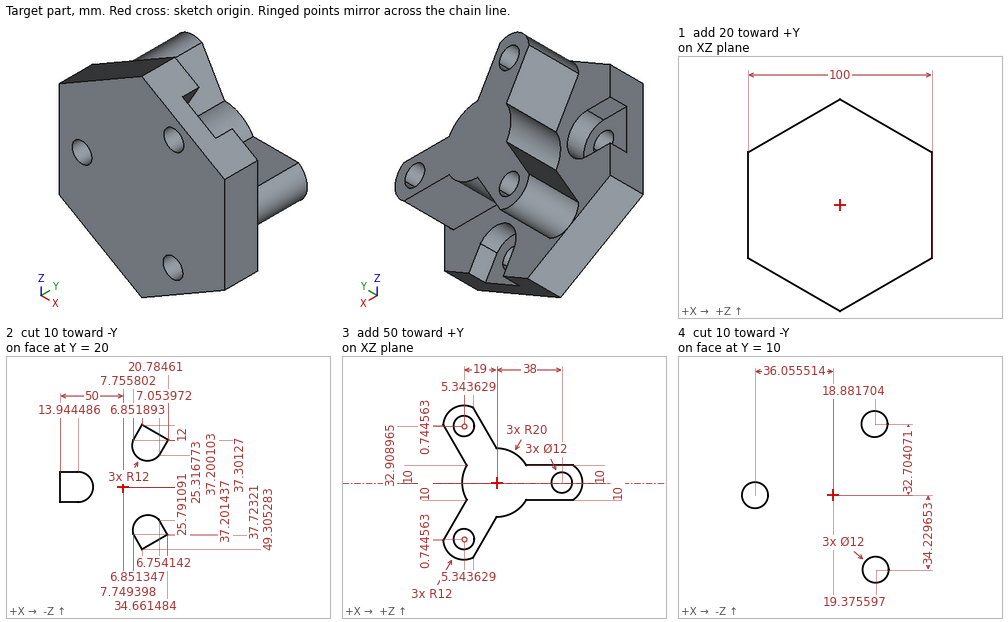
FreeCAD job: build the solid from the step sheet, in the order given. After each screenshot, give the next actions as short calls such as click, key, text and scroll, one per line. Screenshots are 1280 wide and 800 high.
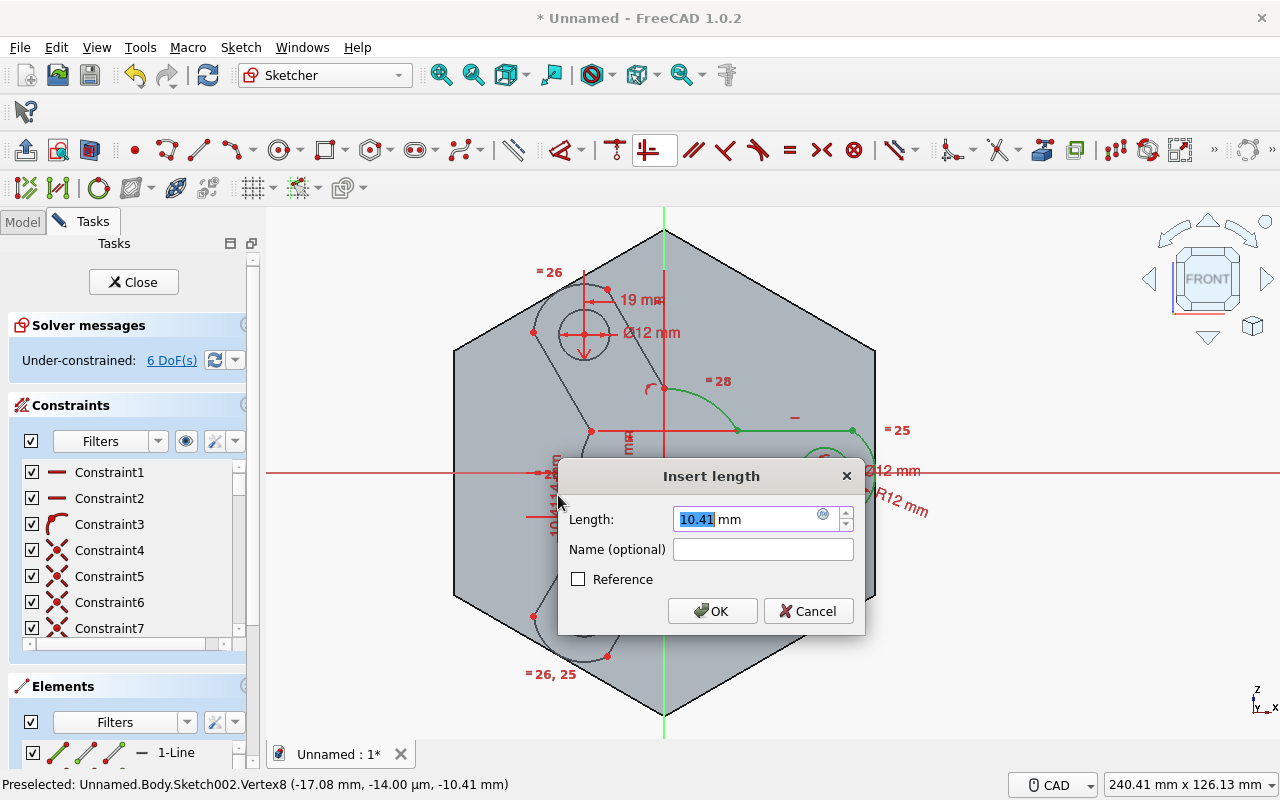
text(10)
key(Return)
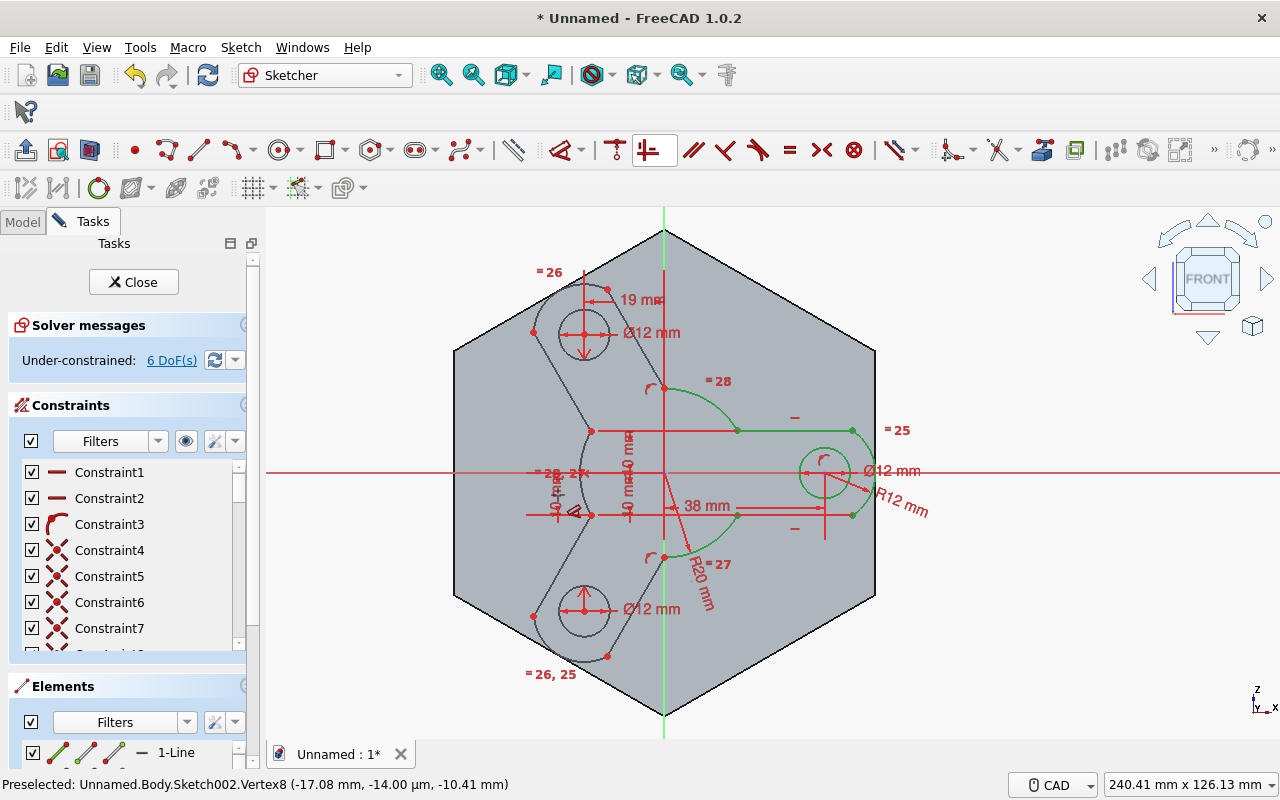
click(591, 432)
click(557, 452)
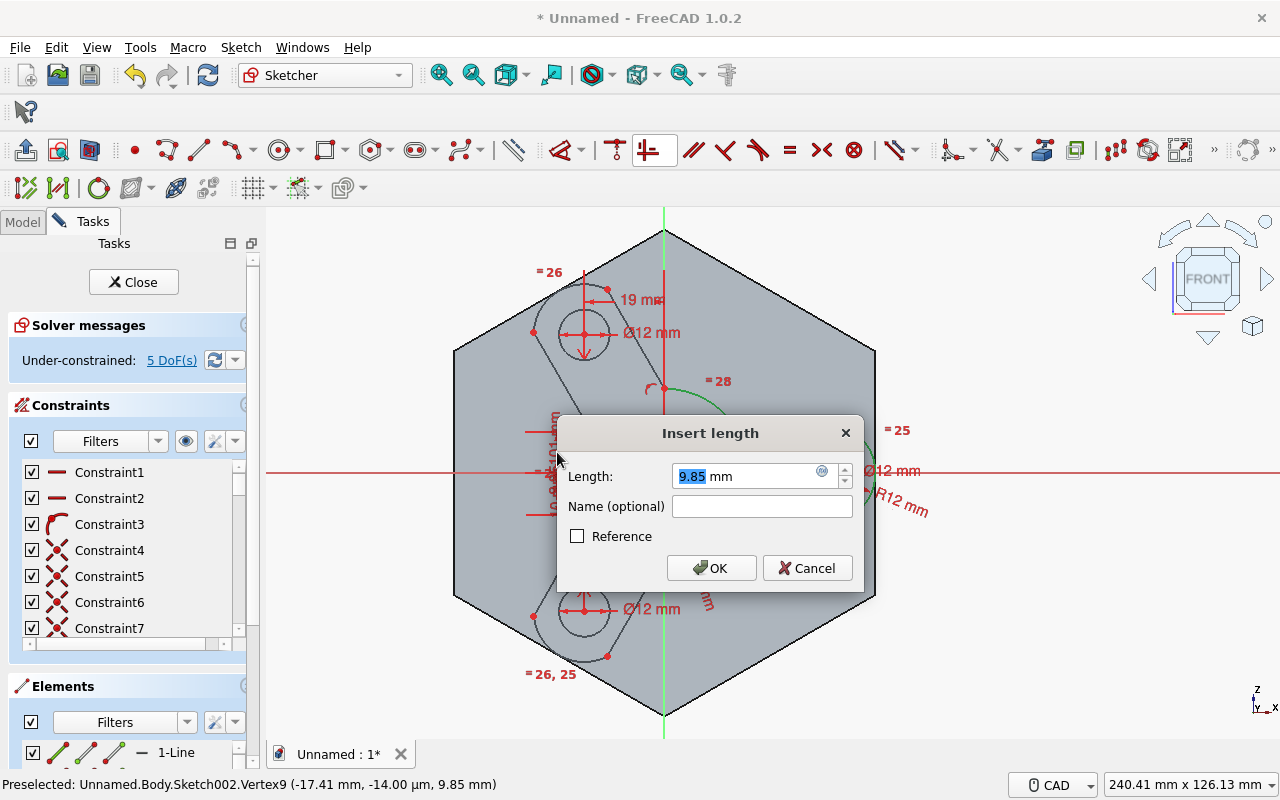
text(10)
key(Return)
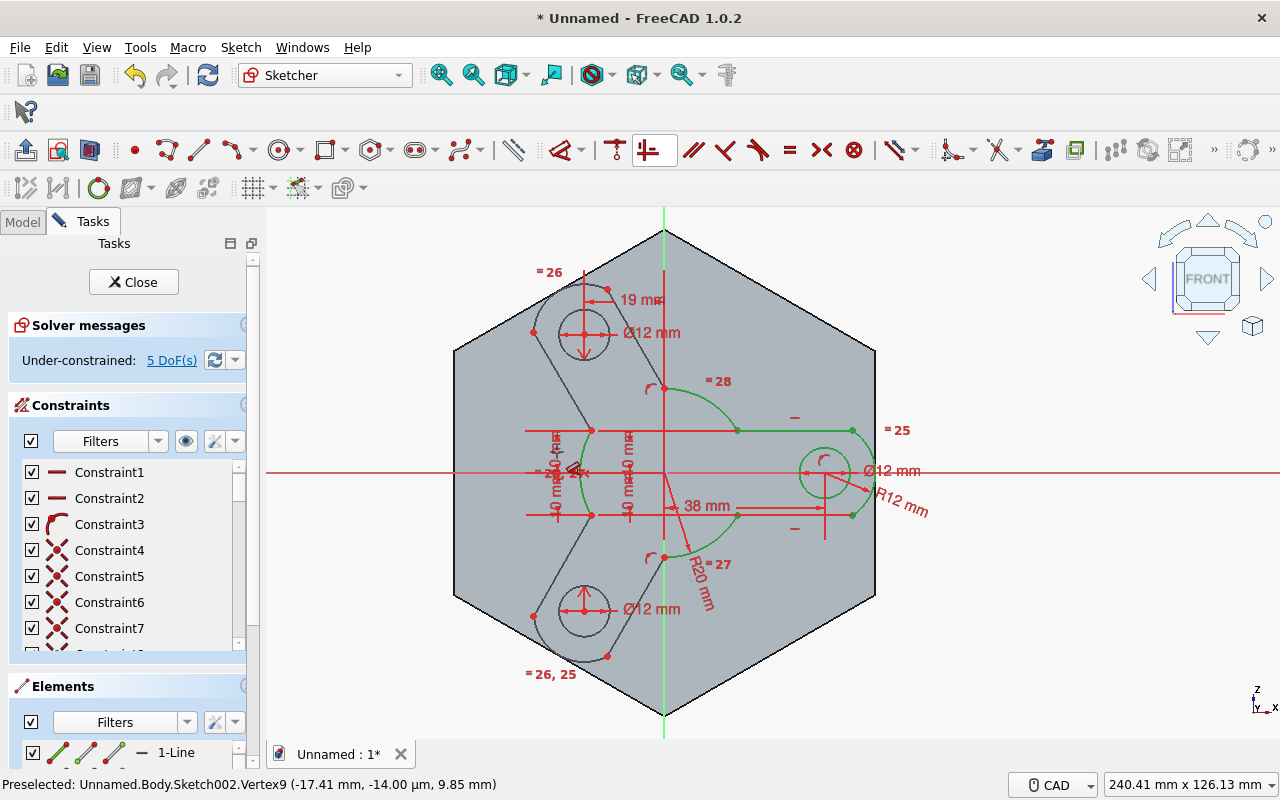
click(584, 335)
click(550, 404)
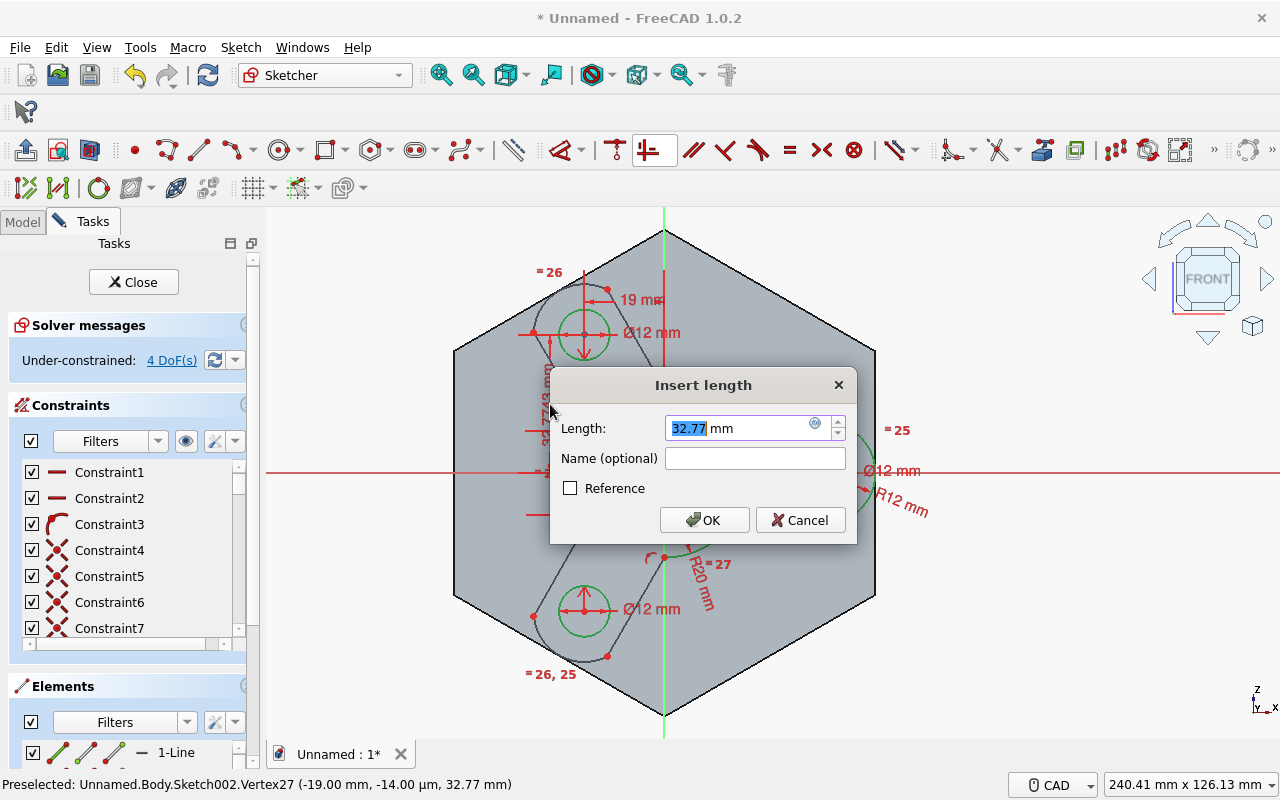
text(32.908965)
key(Return)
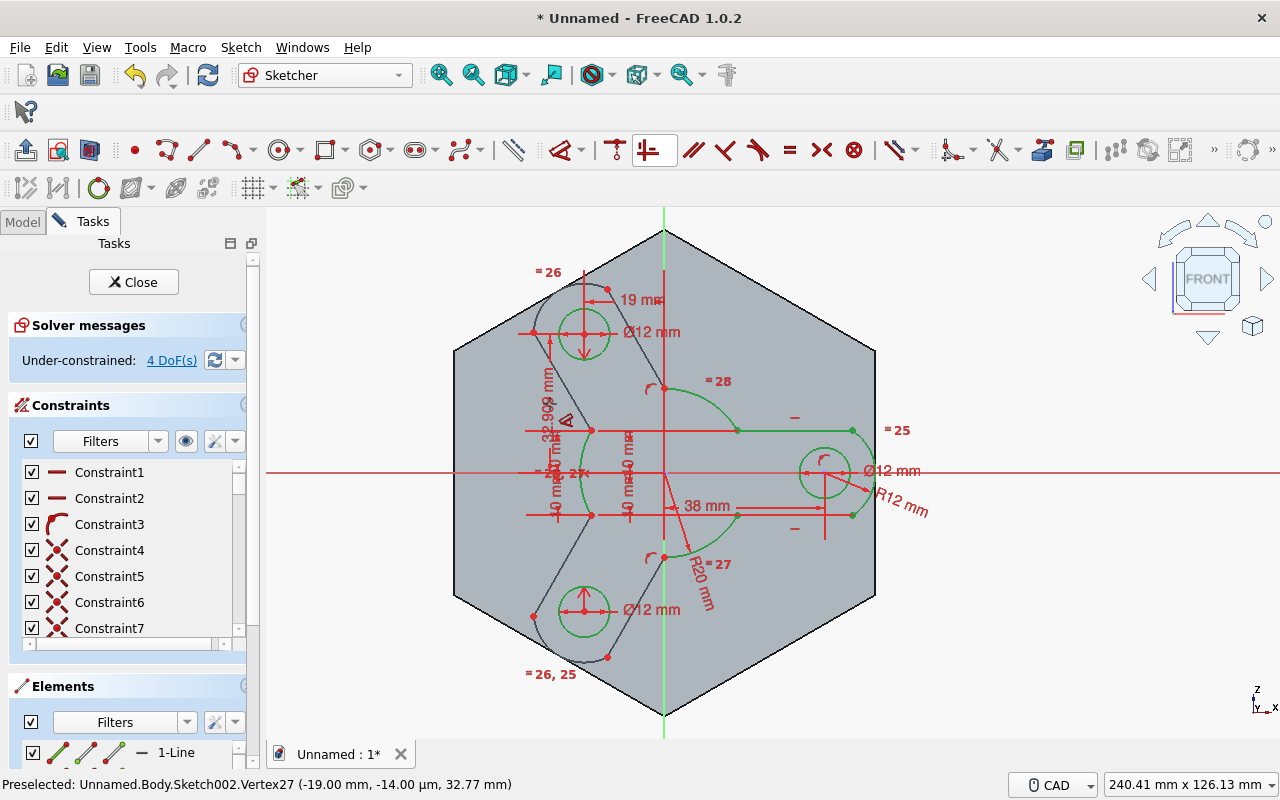
scroll(607, 289, up, 3)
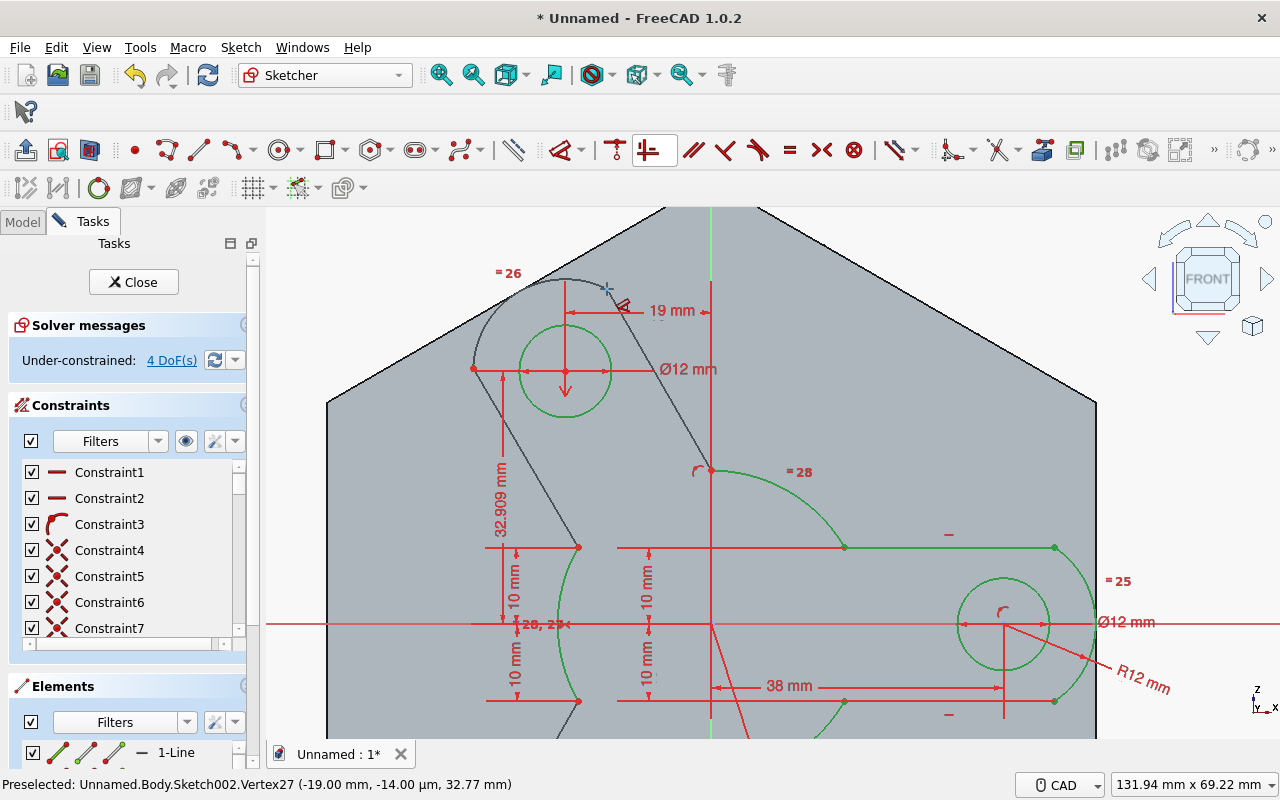
click(607, 289)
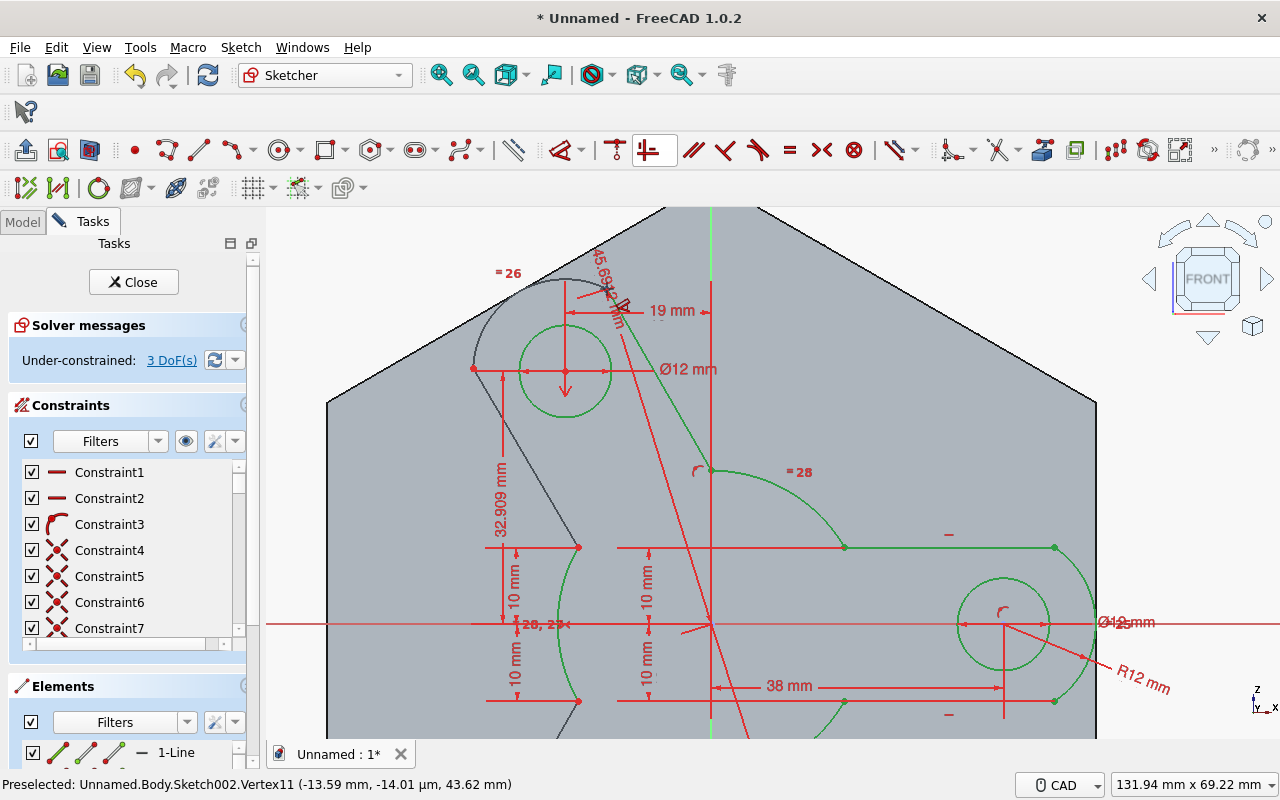
click(565, 371)
click(586, 255)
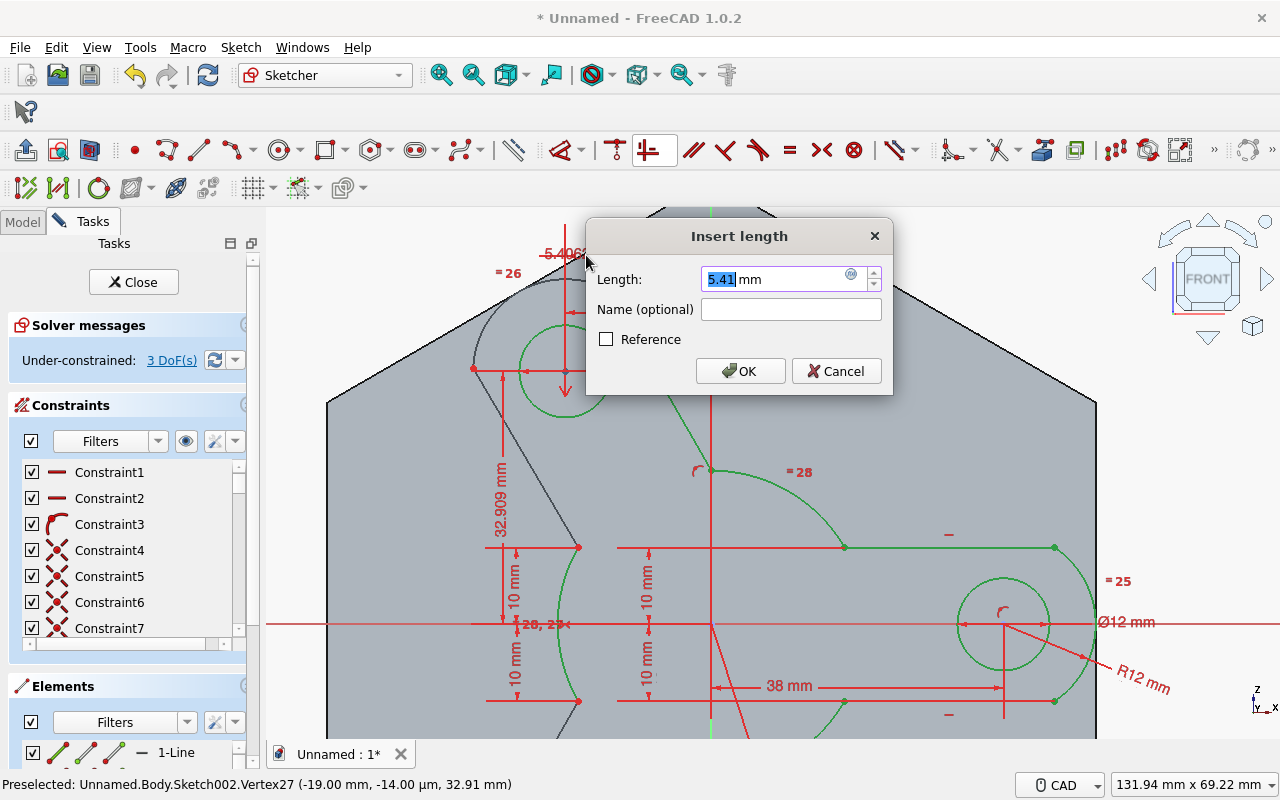
text(5.343629)
key(Return)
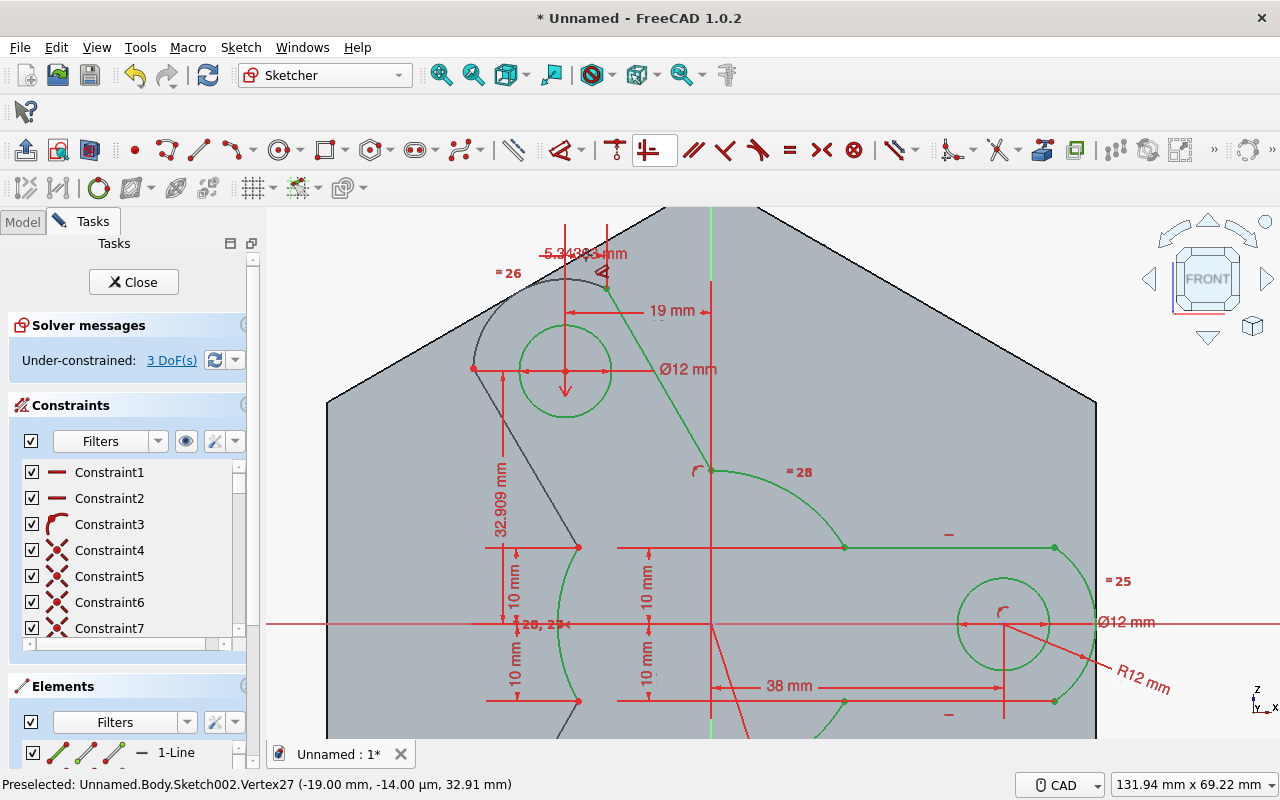
scroll(473, 368, up, 10)